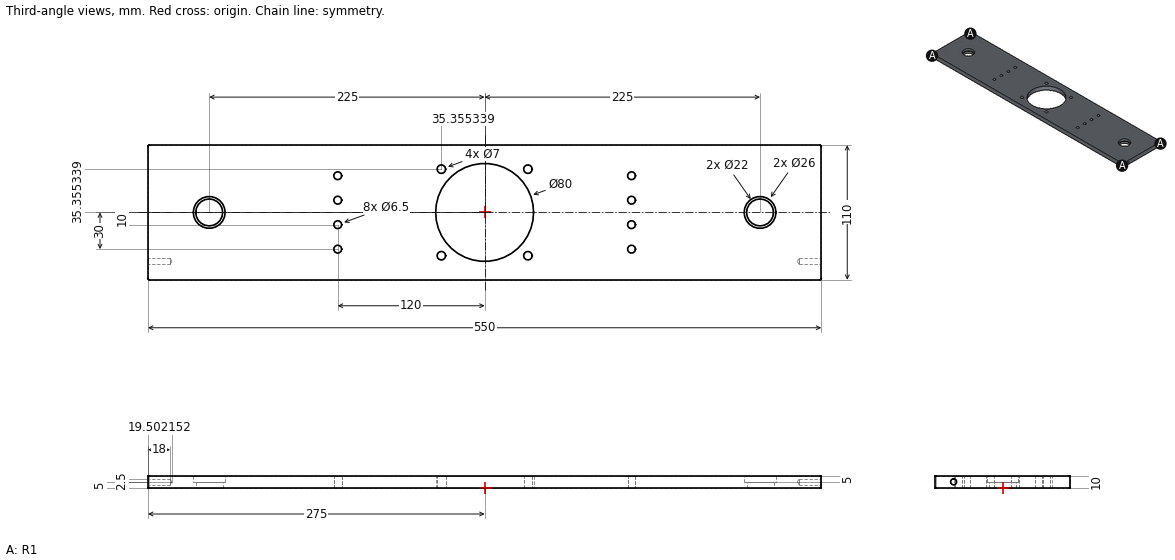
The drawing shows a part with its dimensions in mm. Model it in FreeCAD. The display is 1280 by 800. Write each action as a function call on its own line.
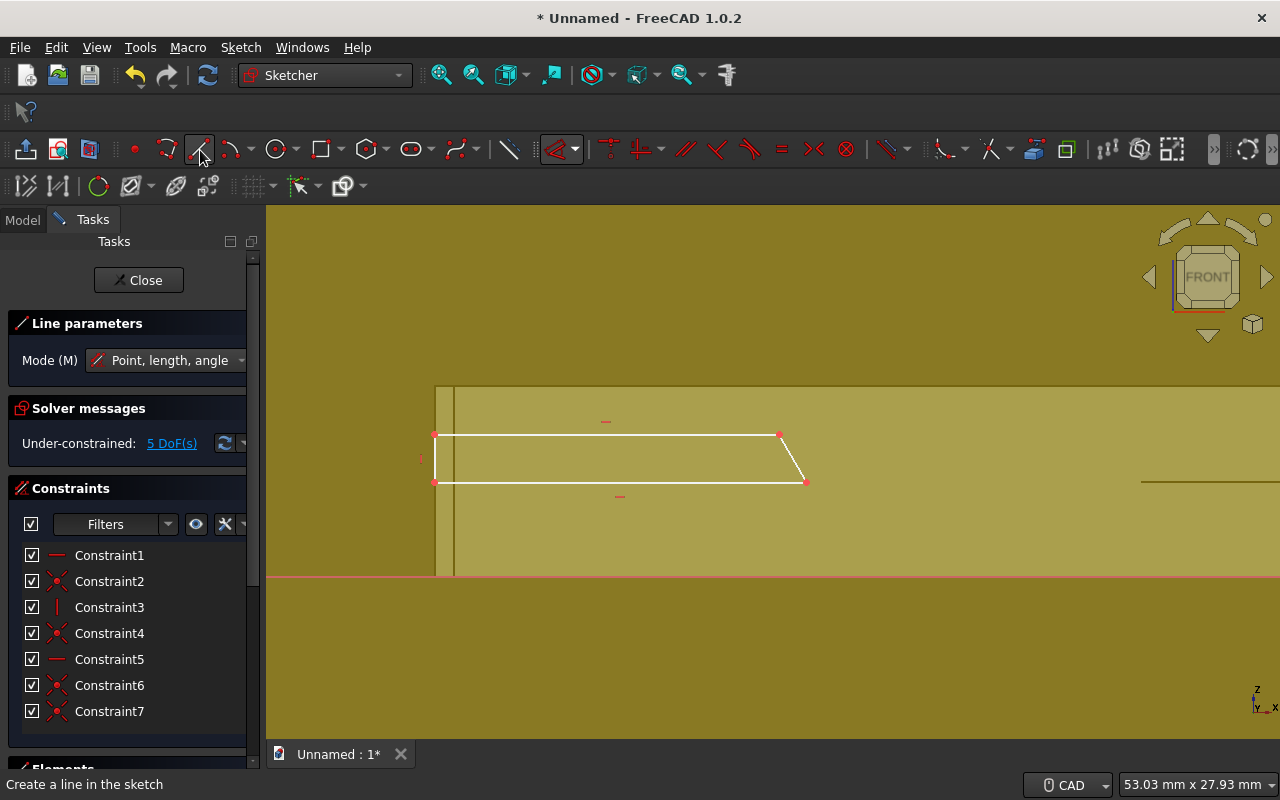
click(845, 482)
click(957, 482)
key(Escape)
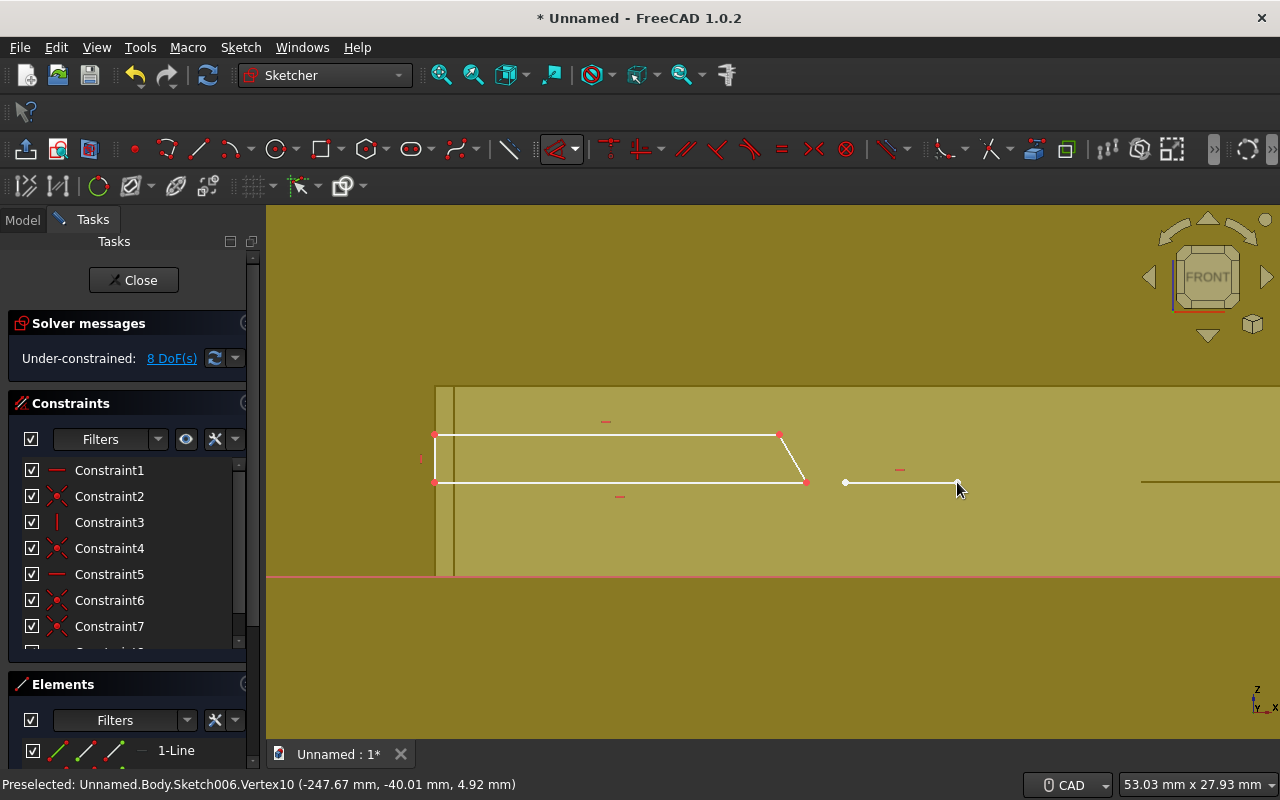
click(879, 483)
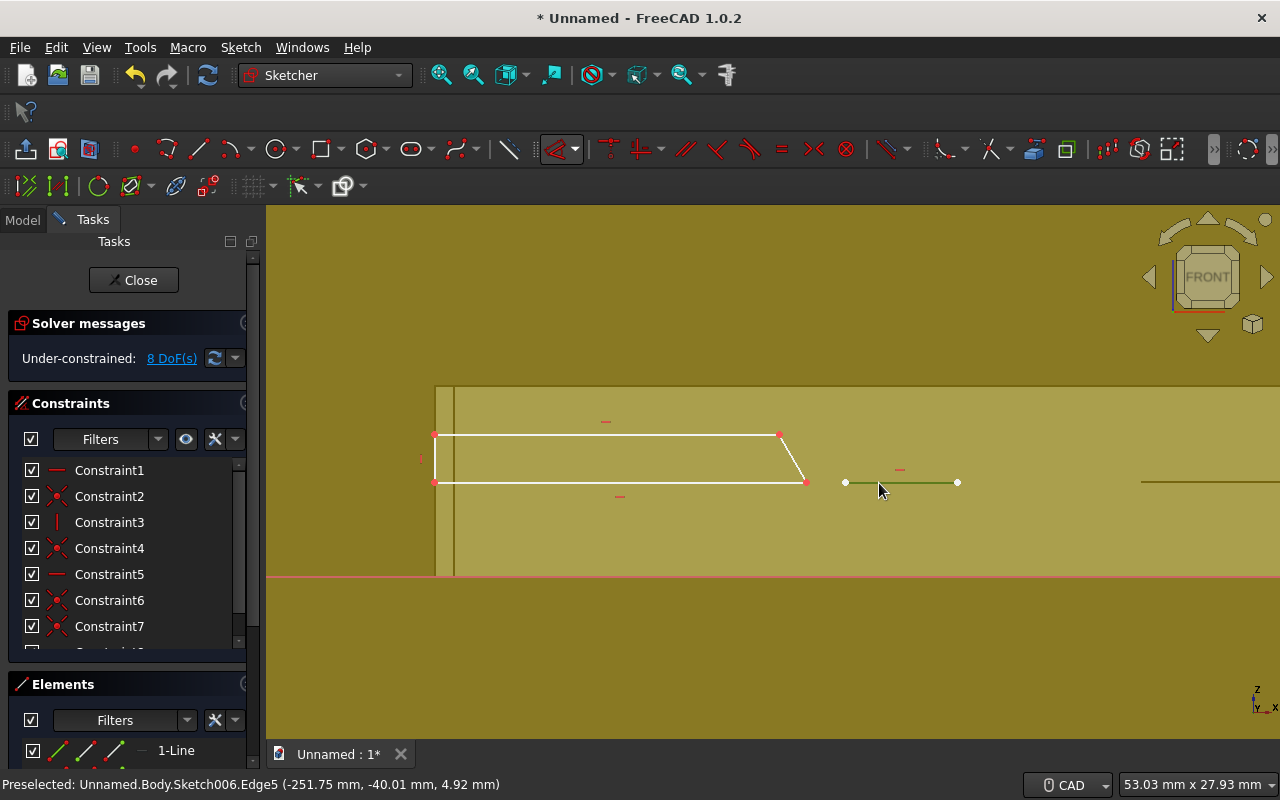
key(g)
key(n)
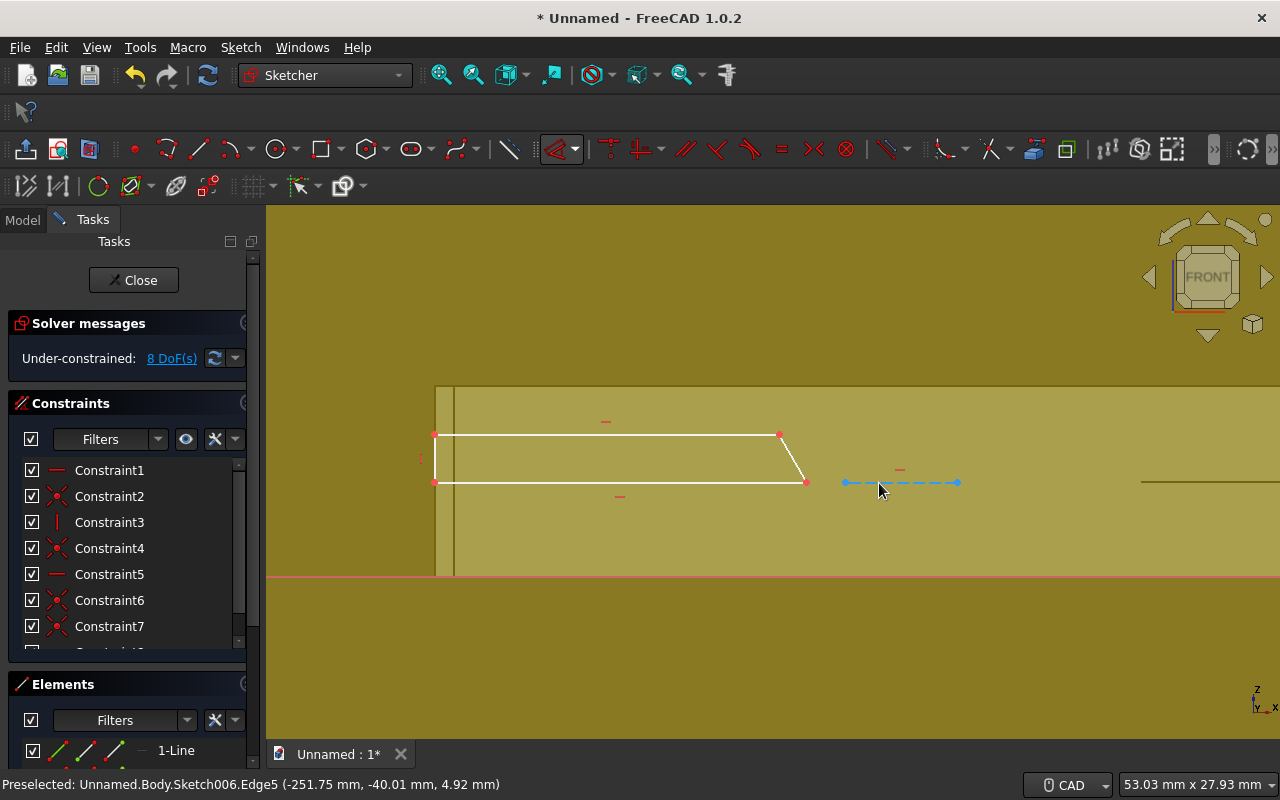
click(538, 435)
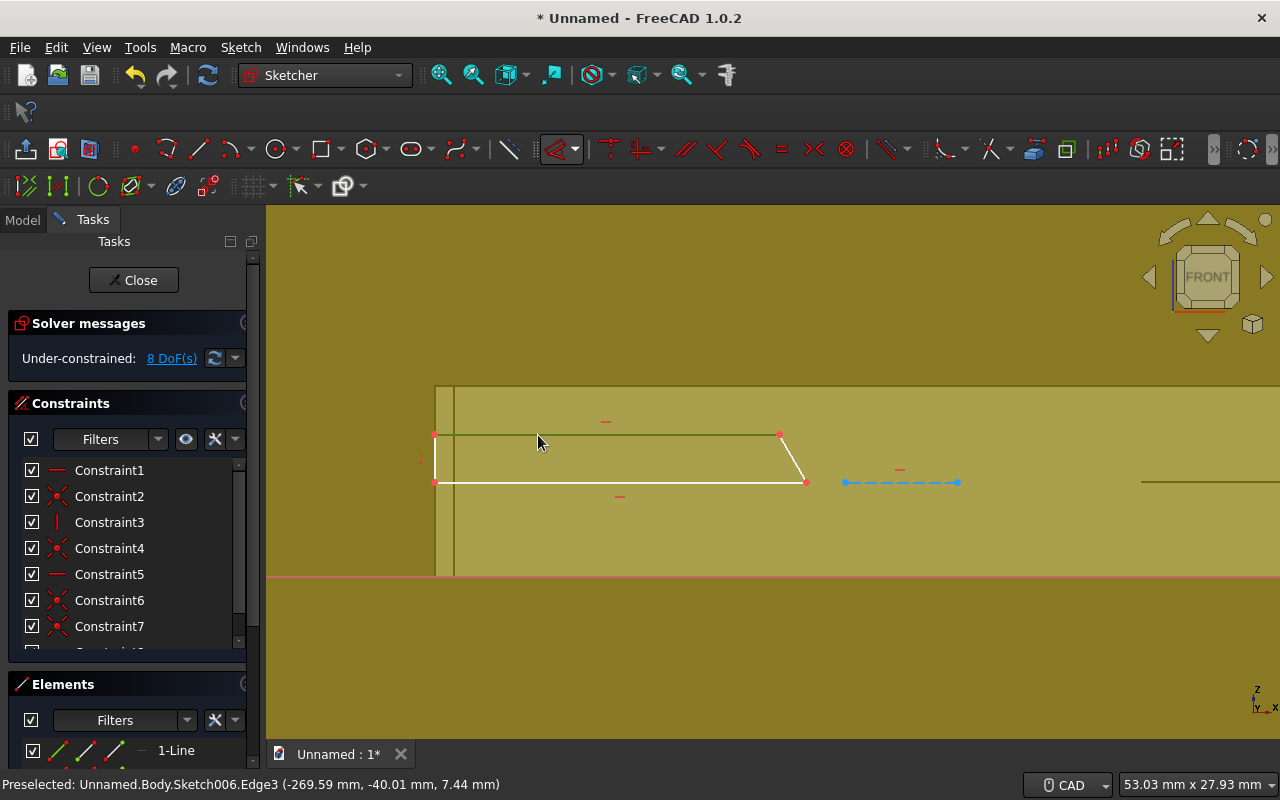
click(578, 150)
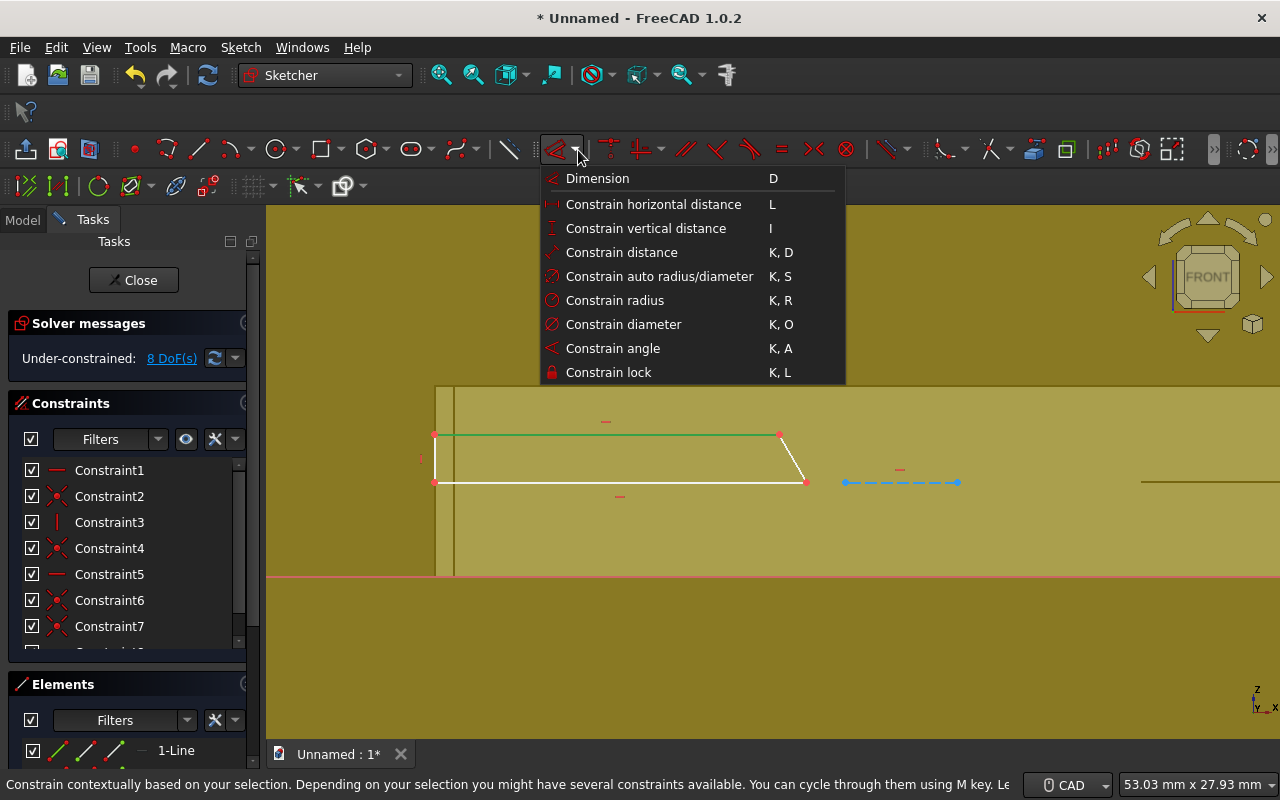
click(693, 204)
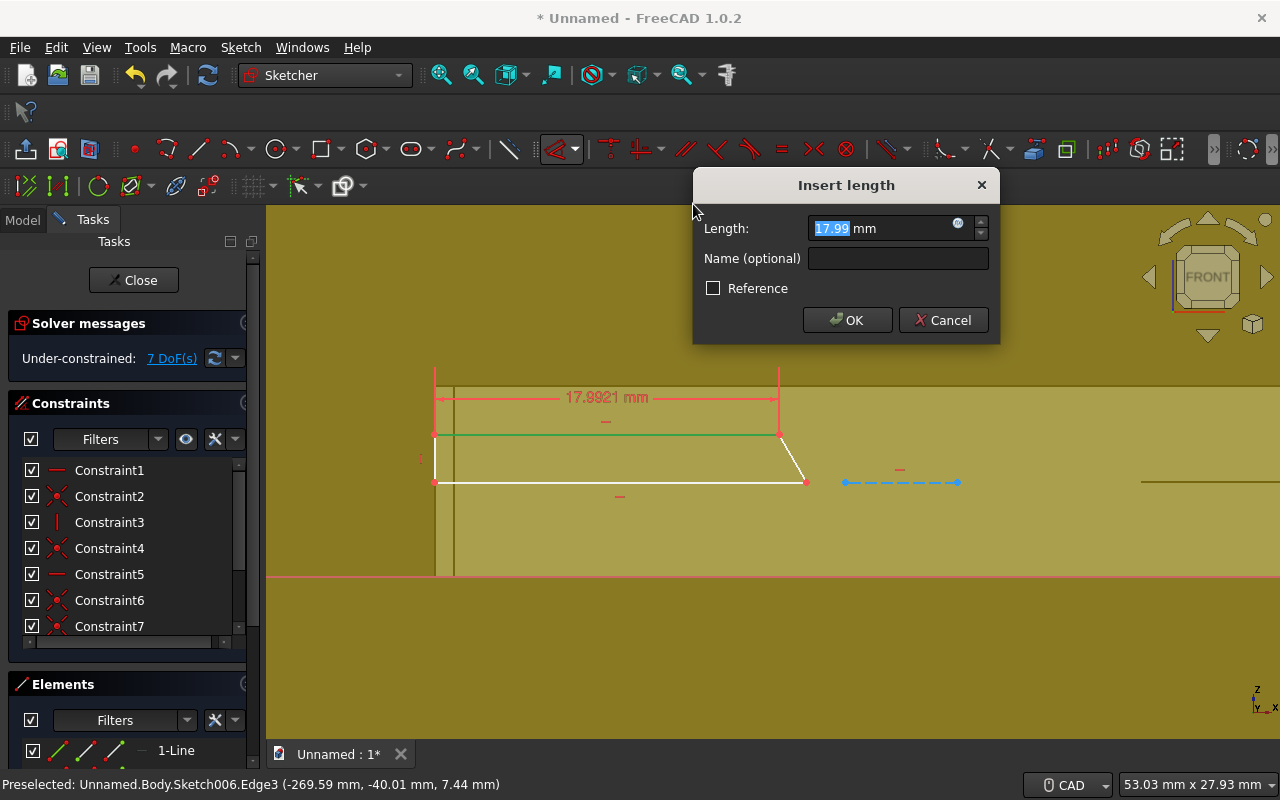
text(18)
key(Return)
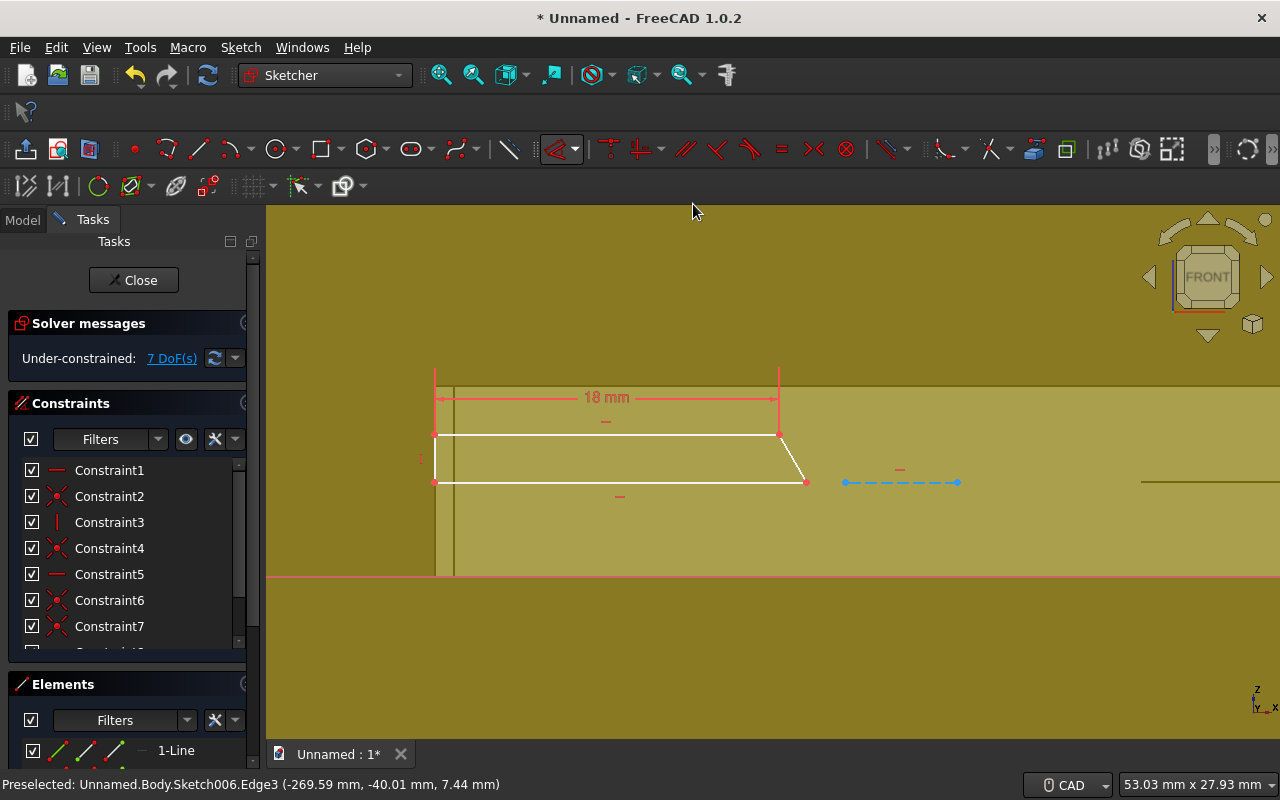
click(807, 483)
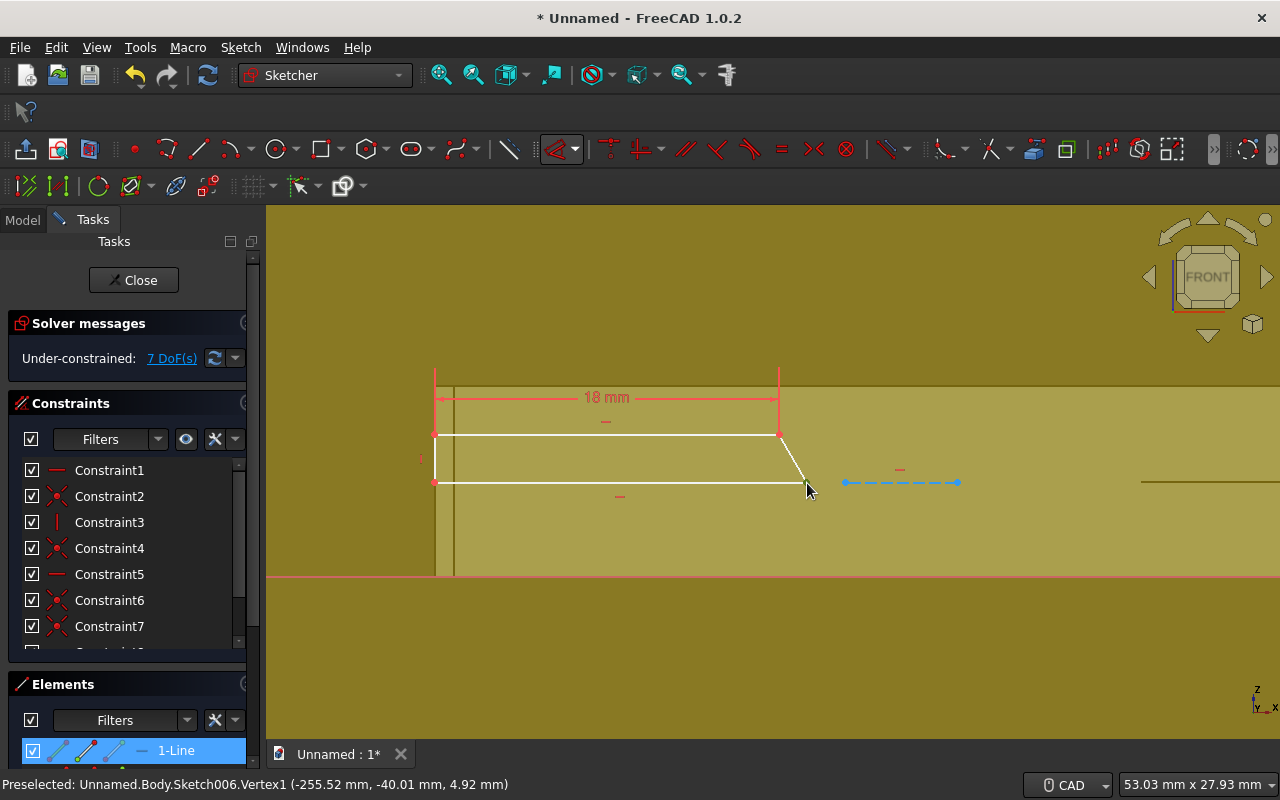
key(i)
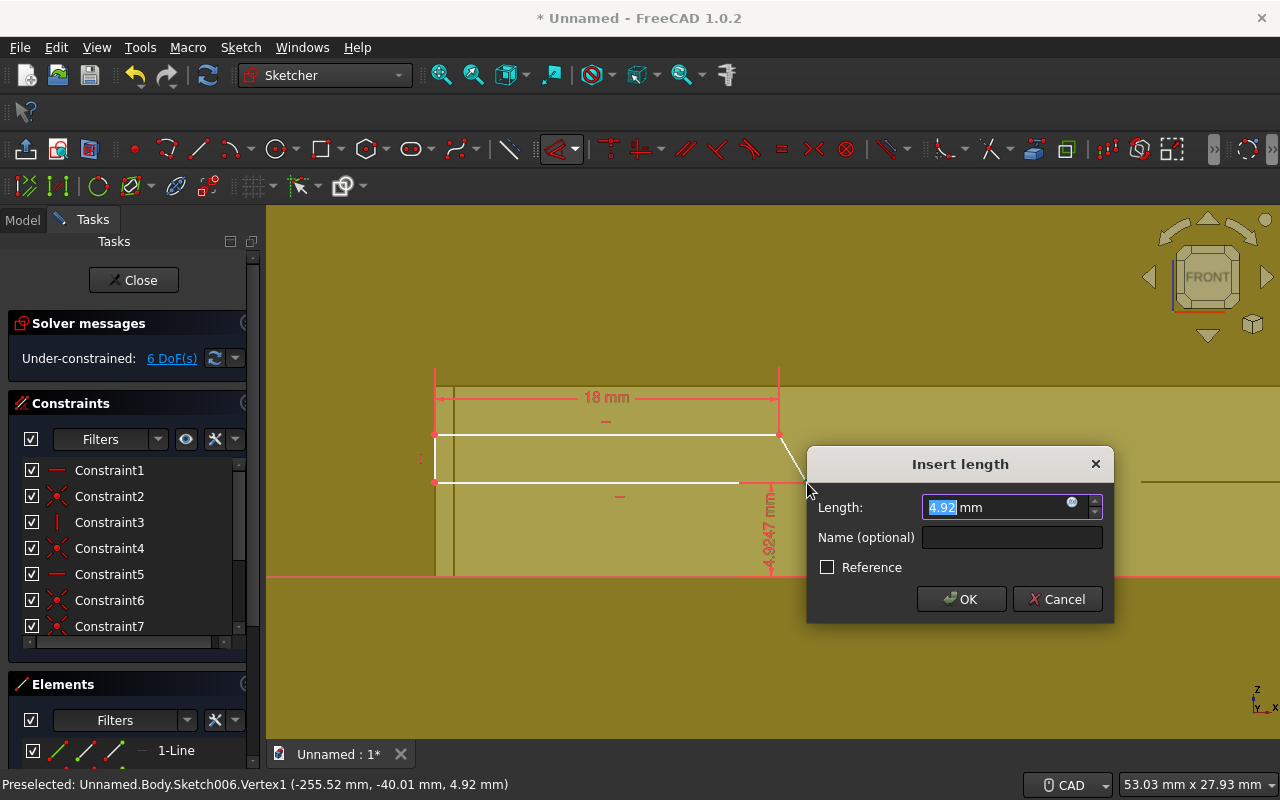
text(5)
key(Return)